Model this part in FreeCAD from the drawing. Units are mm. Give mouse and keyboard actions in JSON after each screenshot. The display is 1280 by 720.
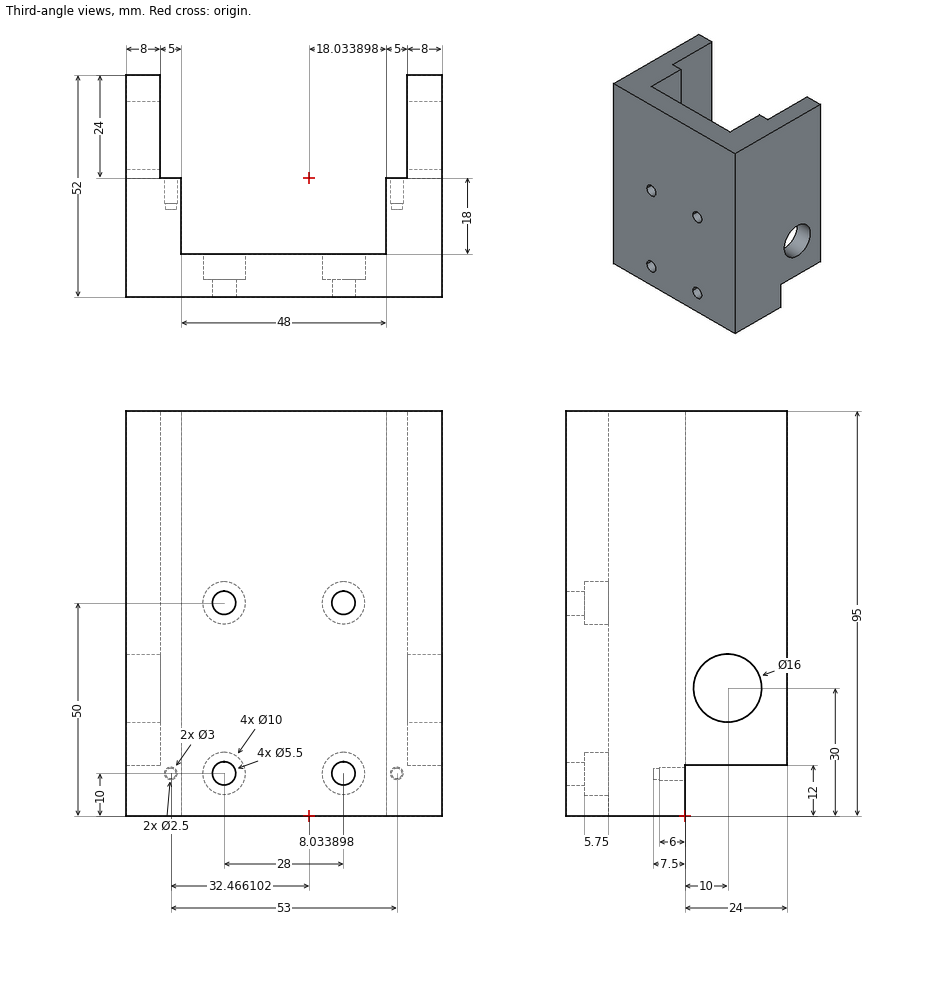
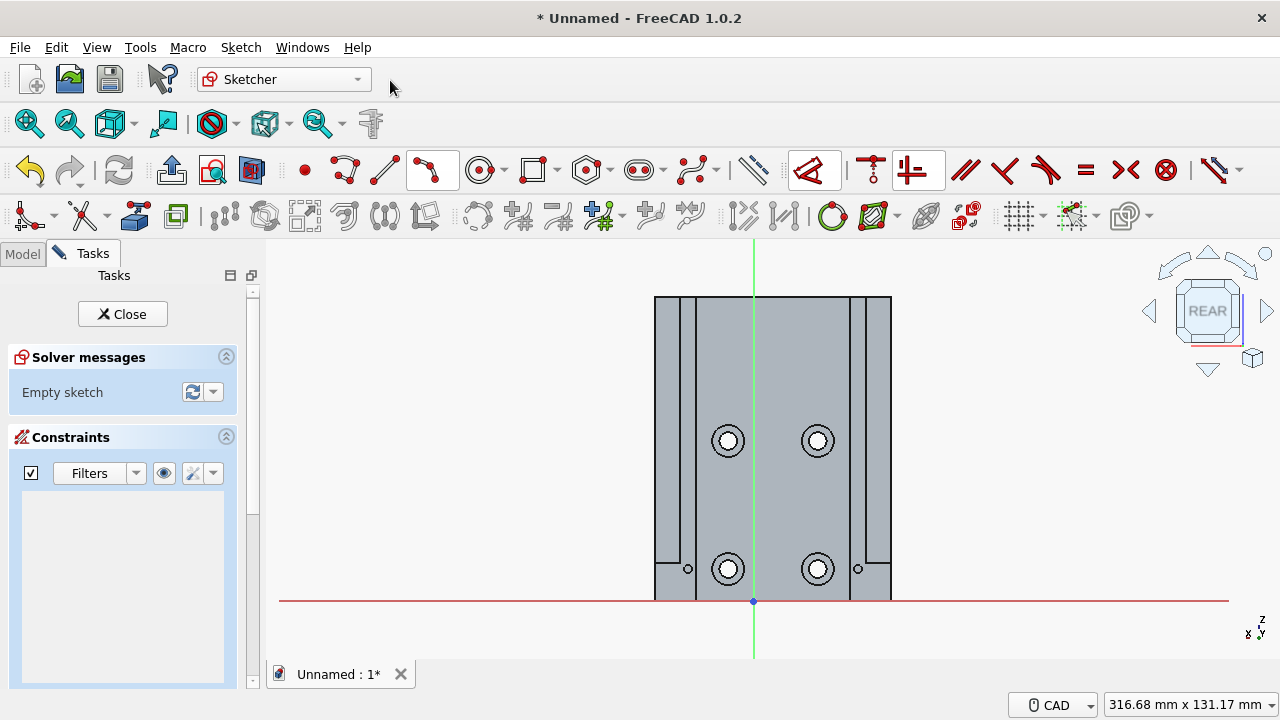
{"action": "scroll", "coordinate": [803, 631], "scroll_direction": "up", "scroll_amount": 6}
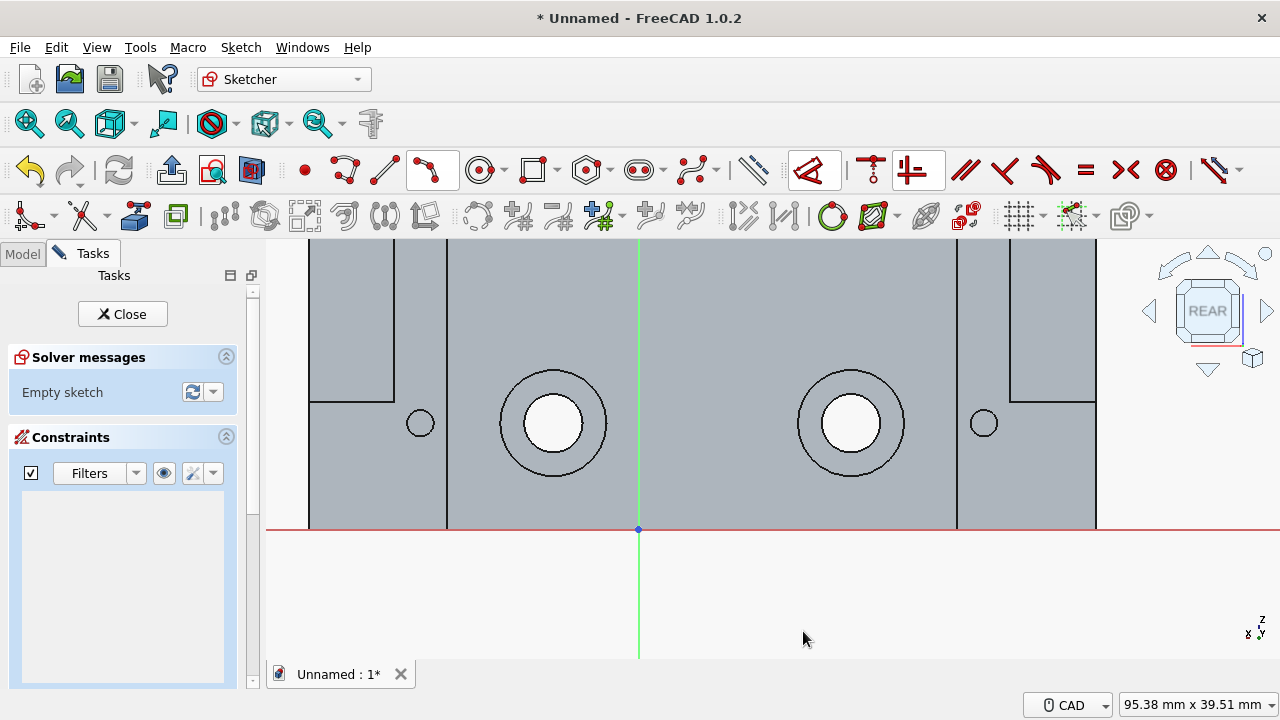
{"action": "left_click", "coordinate": [480, 170]}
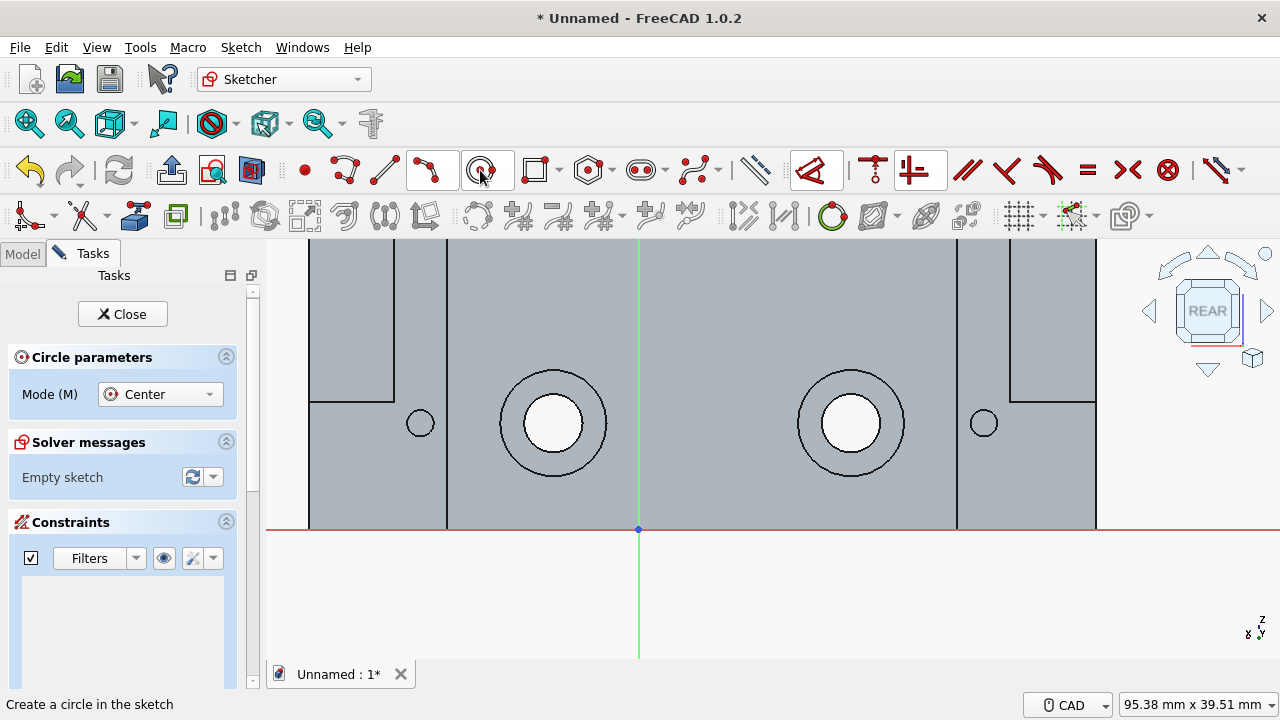
{"action": "scroll", "coordinate": [984, 423], "scroll_direction": "up", "scroll_amount": 2}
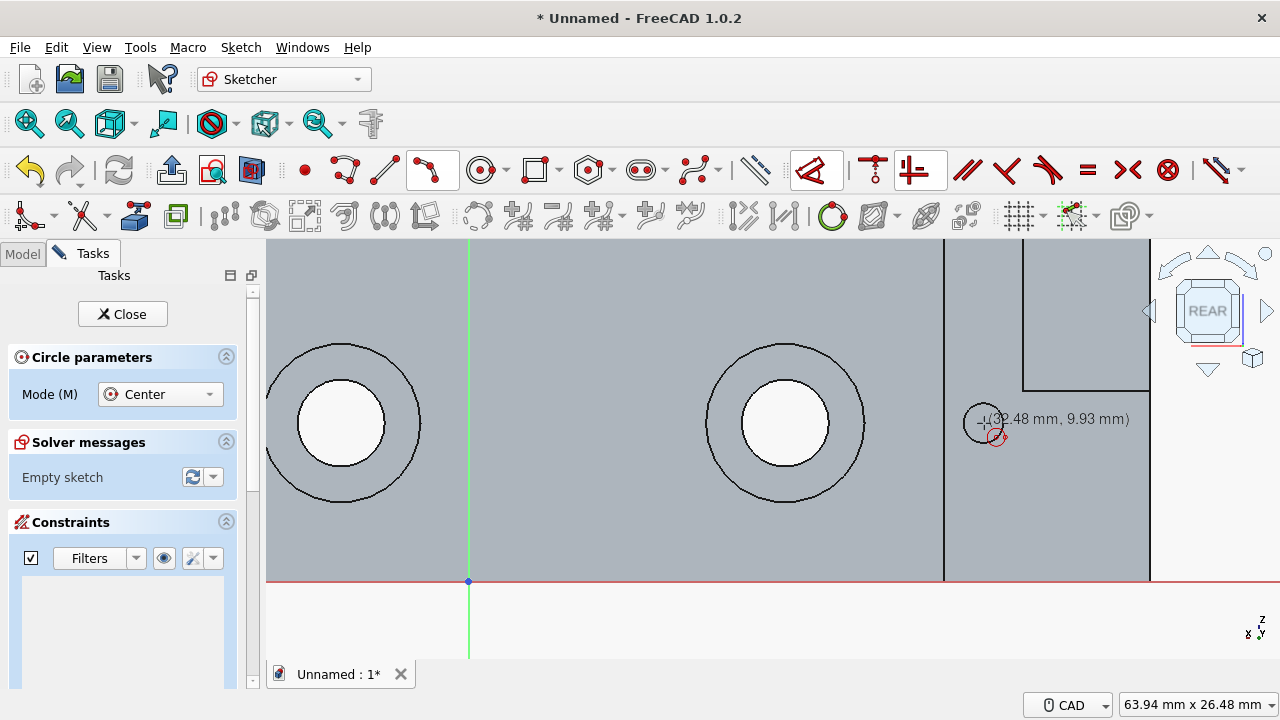
{"action": "left_click", "coordinate": [983, 423]}
{"action": "left_click", "coordinate": [1000, 406]}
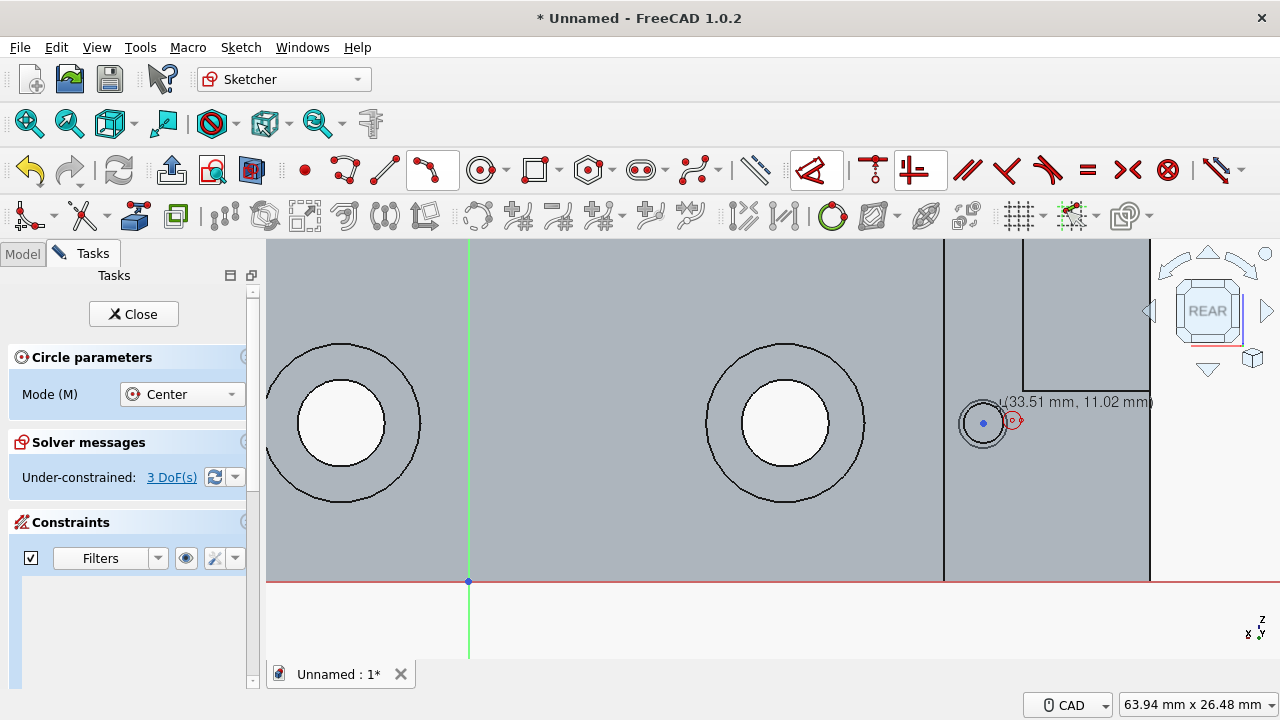
{"action": "scroll", "coordinate": [992, 365], "scroll_direction": "down", "scroll_amount": 2}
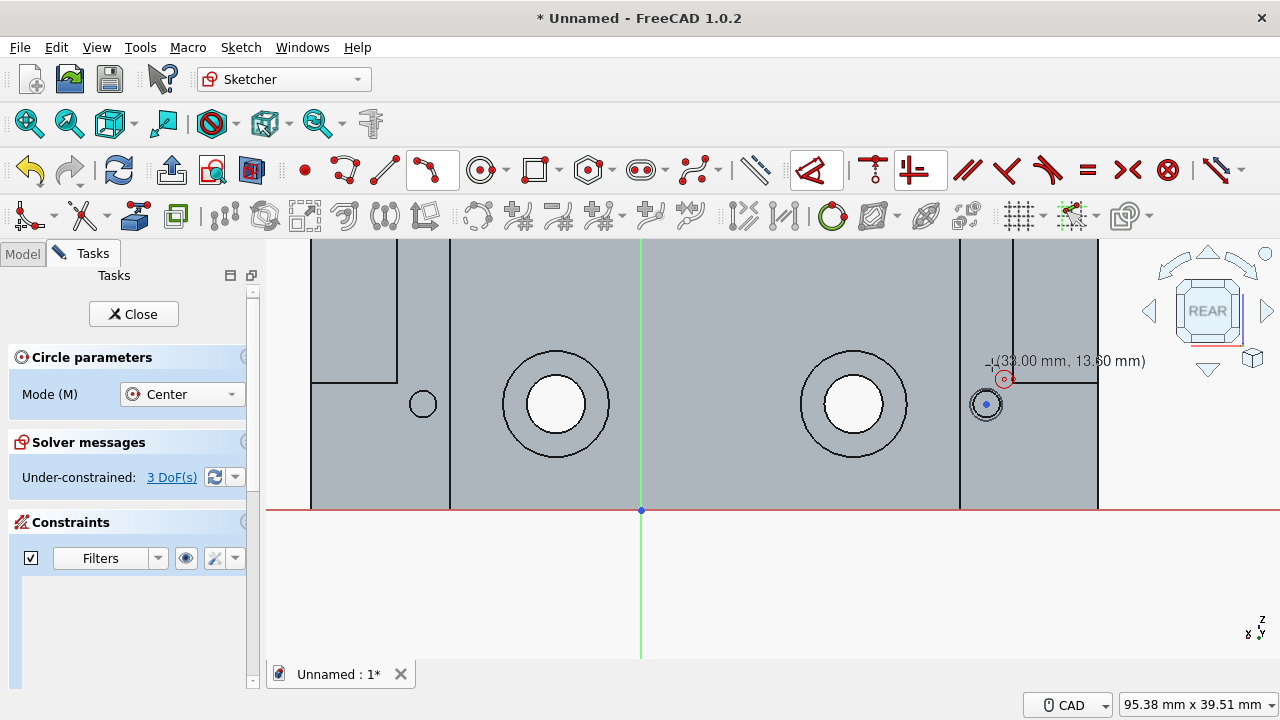
{"action": "scroll", "coordinate": [423, 404], "scroll_direction": "up", "scroll_amount": 2}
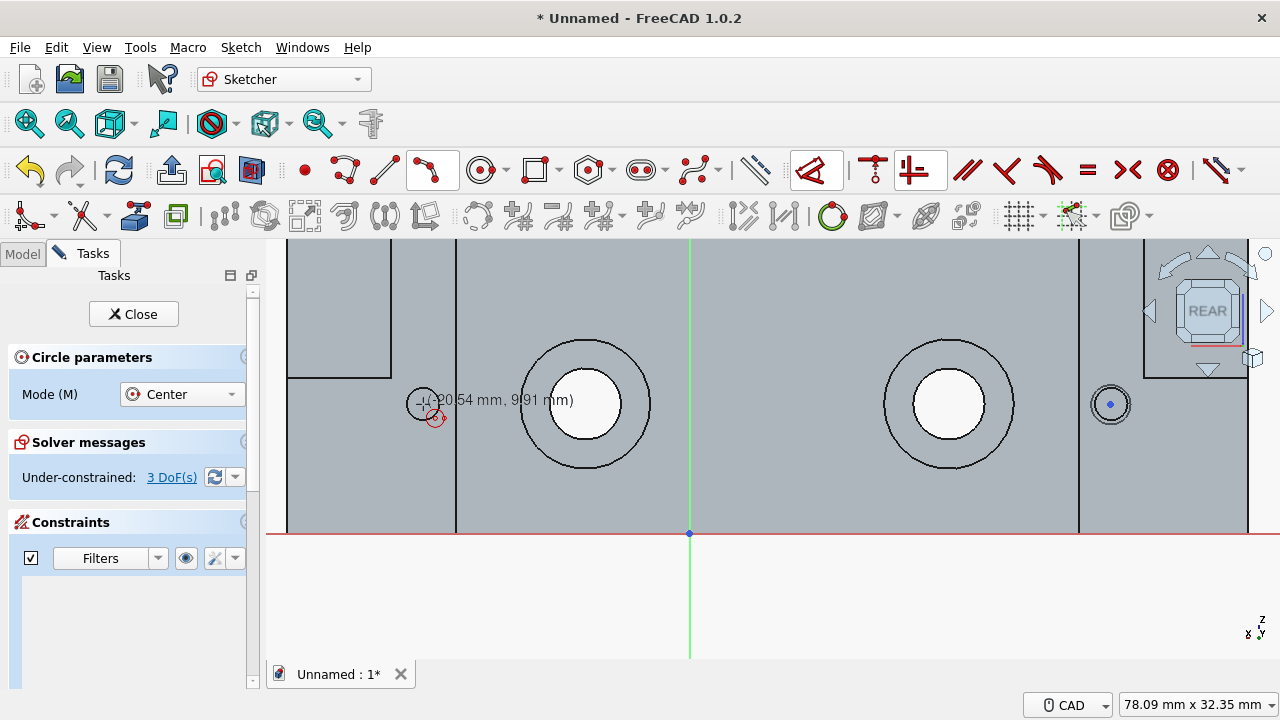
{"action": "left_click", "coordinate": [423, 404]}
{"action": "left_click", "coordinate": [440, 387]}
{"action": "key", "text": "Escape"}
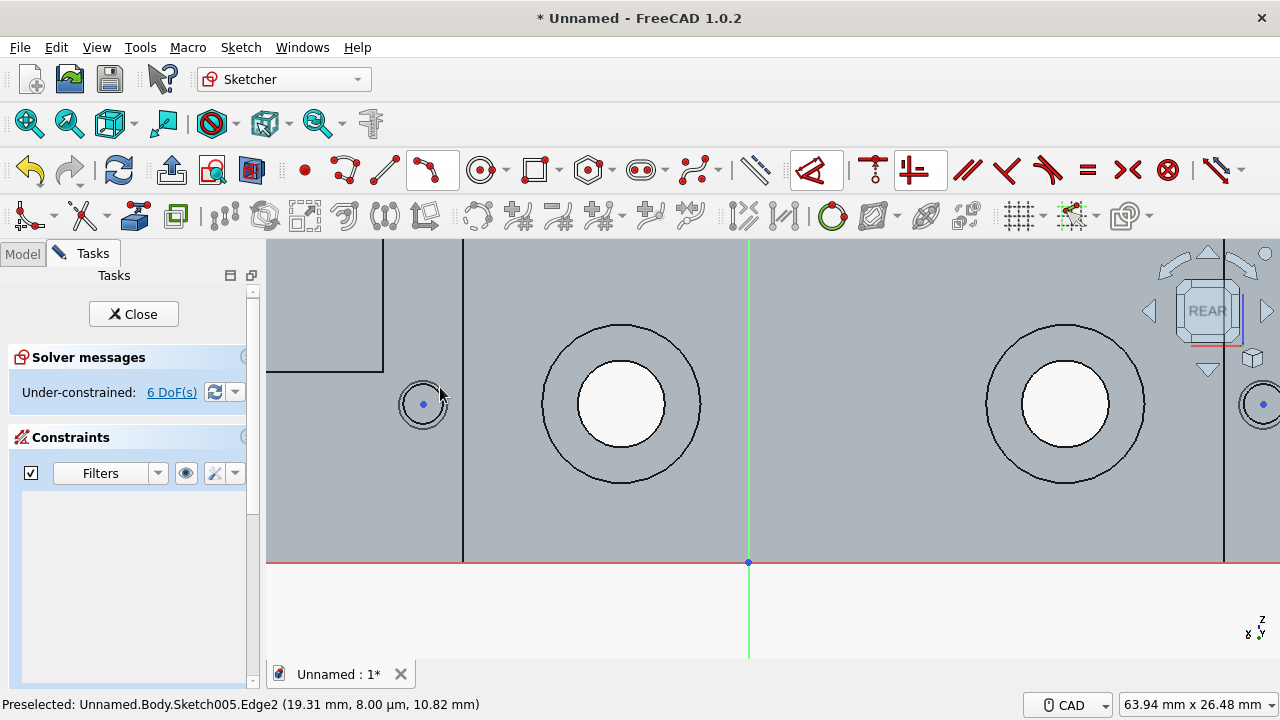
{"action": "scroll", "coordinate": [422, 404], "scroll_direction": "down", "scroll_amount": 2}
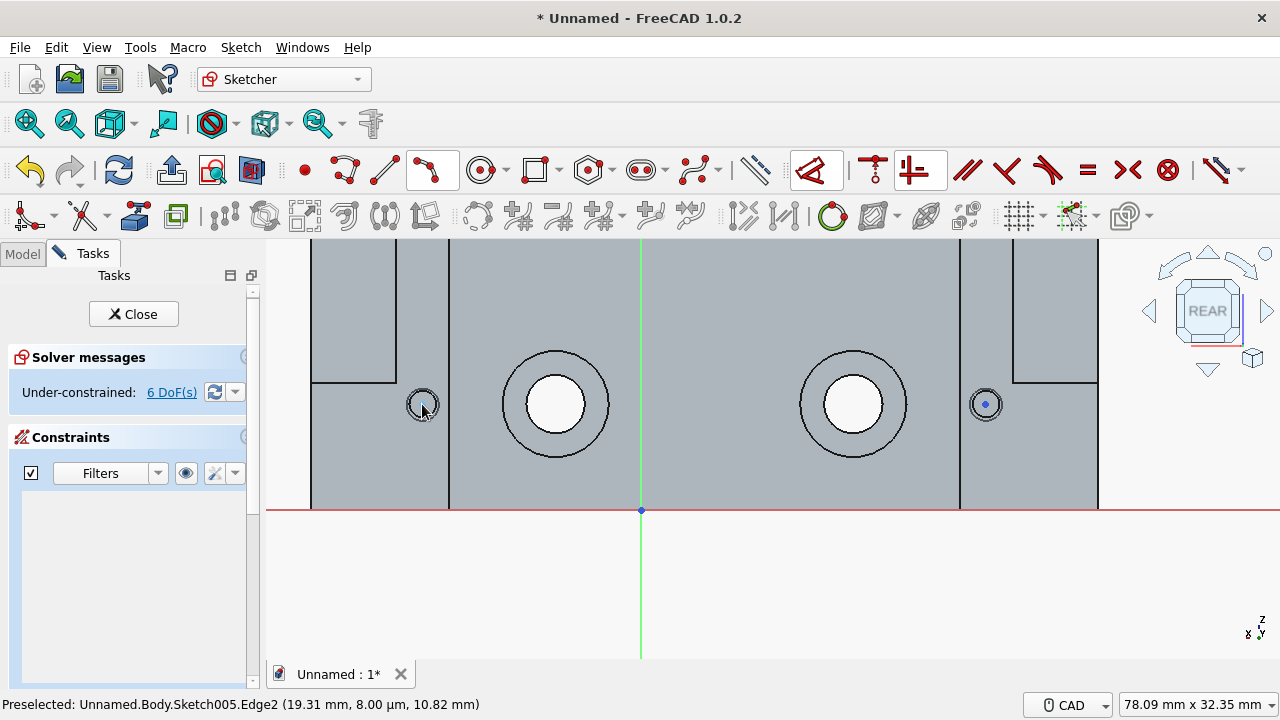
{"action": "left_click", "coordinate": [997, 393]}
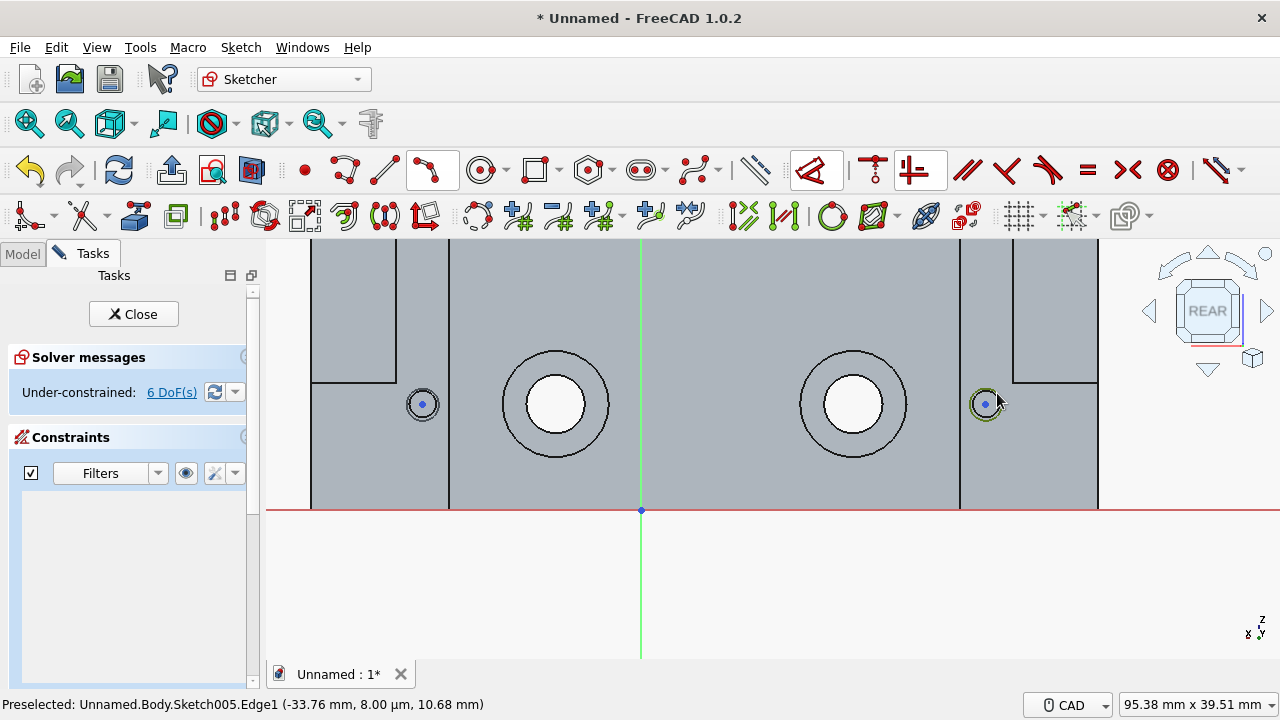
{"action": "left_click", "coordinate": [434, 393]}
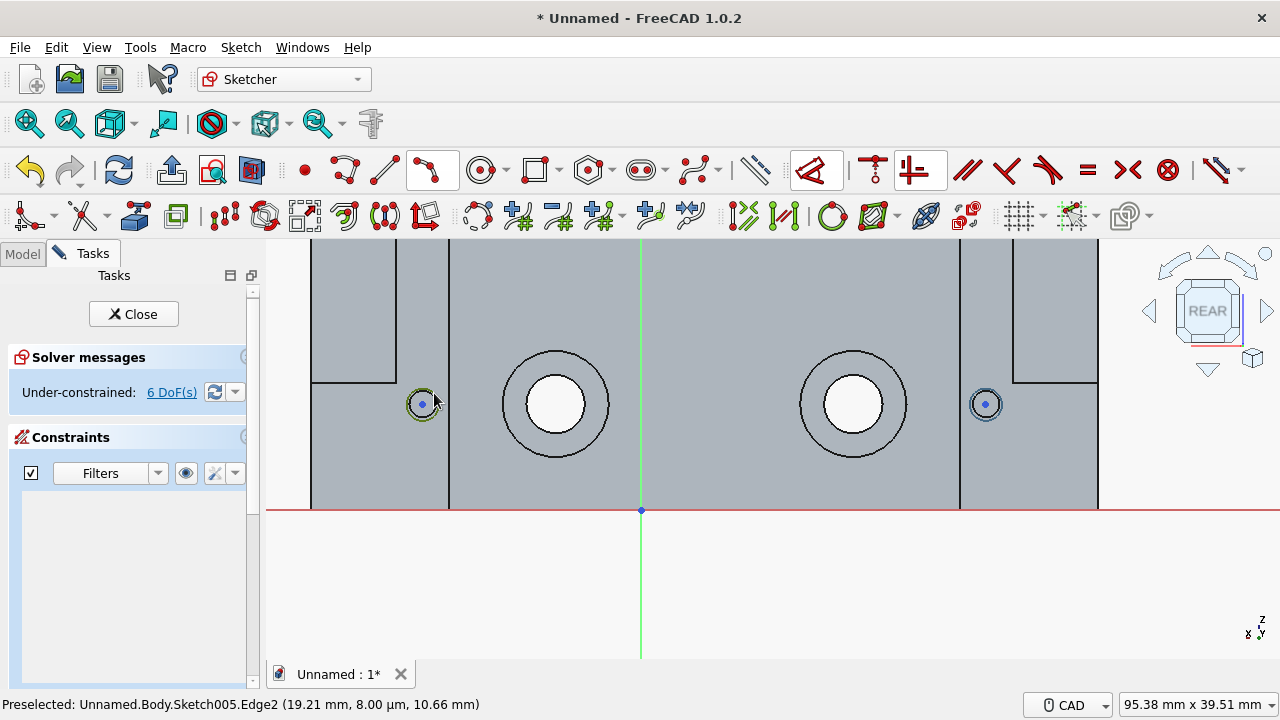
{"action": "key", "text": "e"}